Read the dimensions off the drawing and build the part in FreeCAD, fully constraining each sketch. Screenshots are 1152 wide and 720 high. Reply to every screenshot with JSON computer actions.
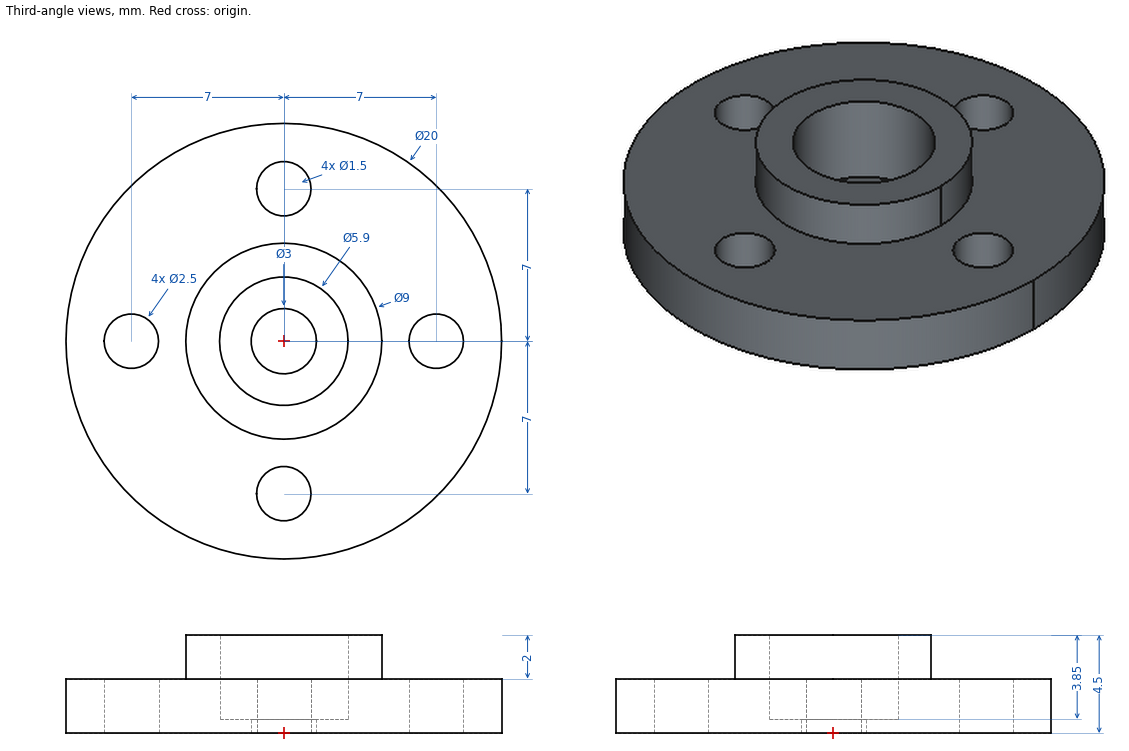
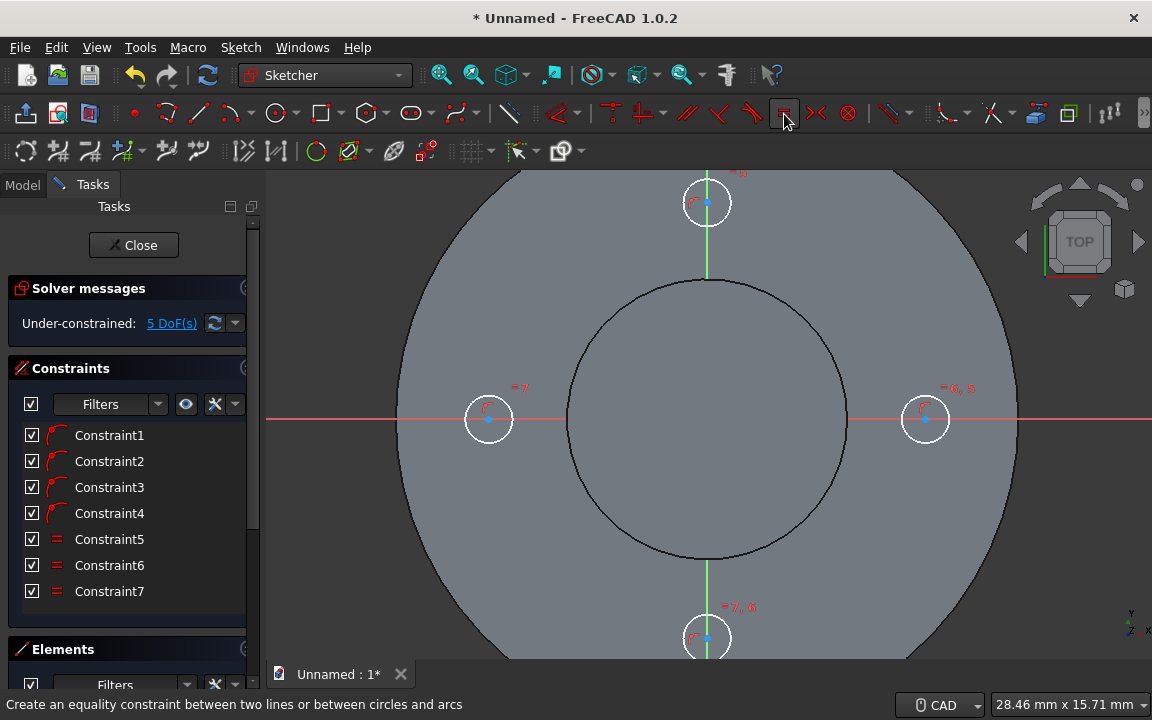
{"action": "left_click", "coordinate": [556, 114]}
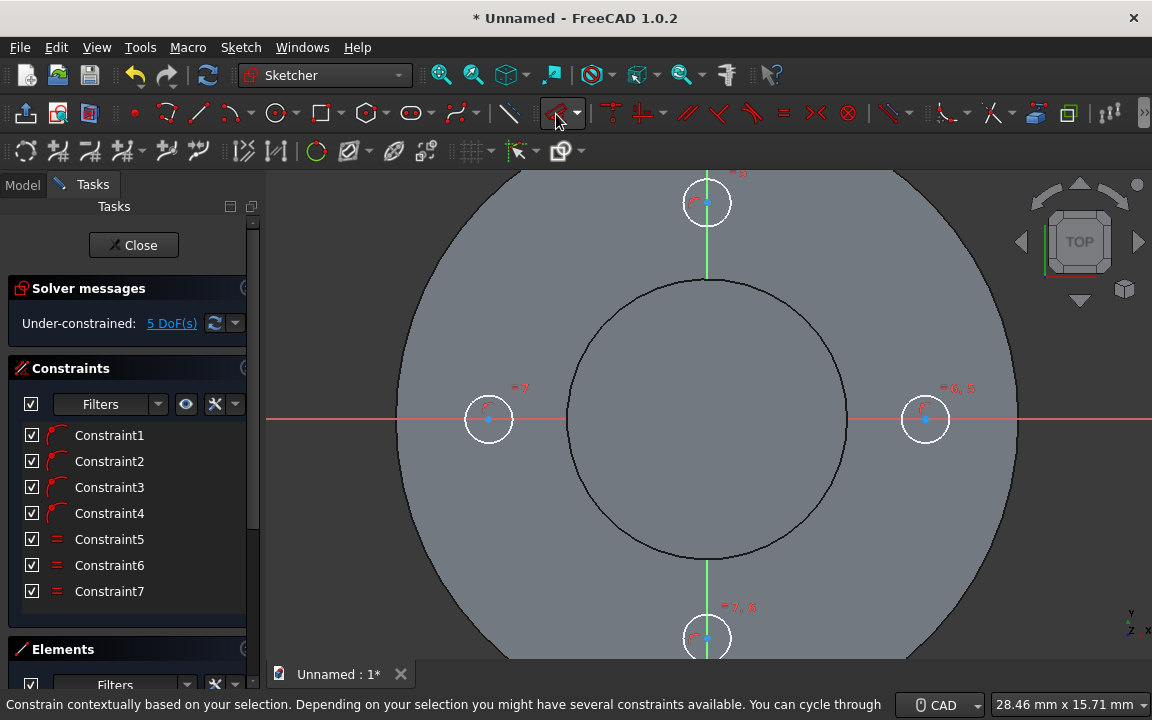
{"action": "left_click", "coordinate": [690, 220]}
{"action": "left_click", "coordinate": [667, 243]}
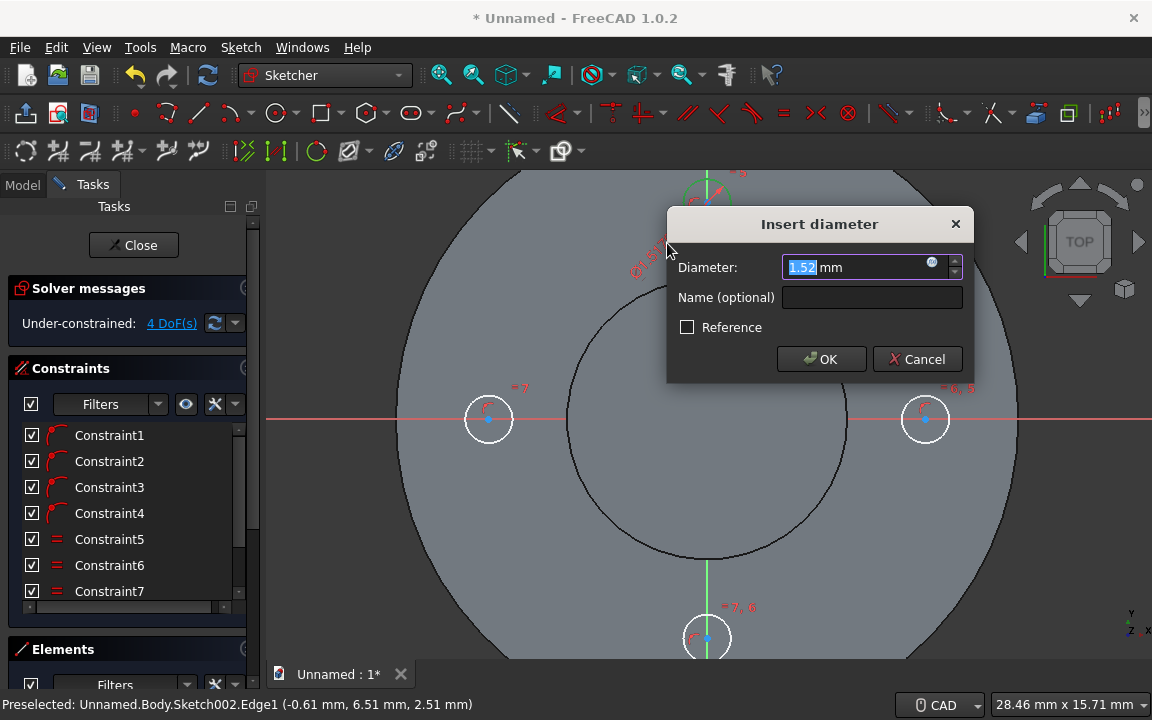
{"action": "type", "text": "1.5"}
{"action": "key", "text": "Return"}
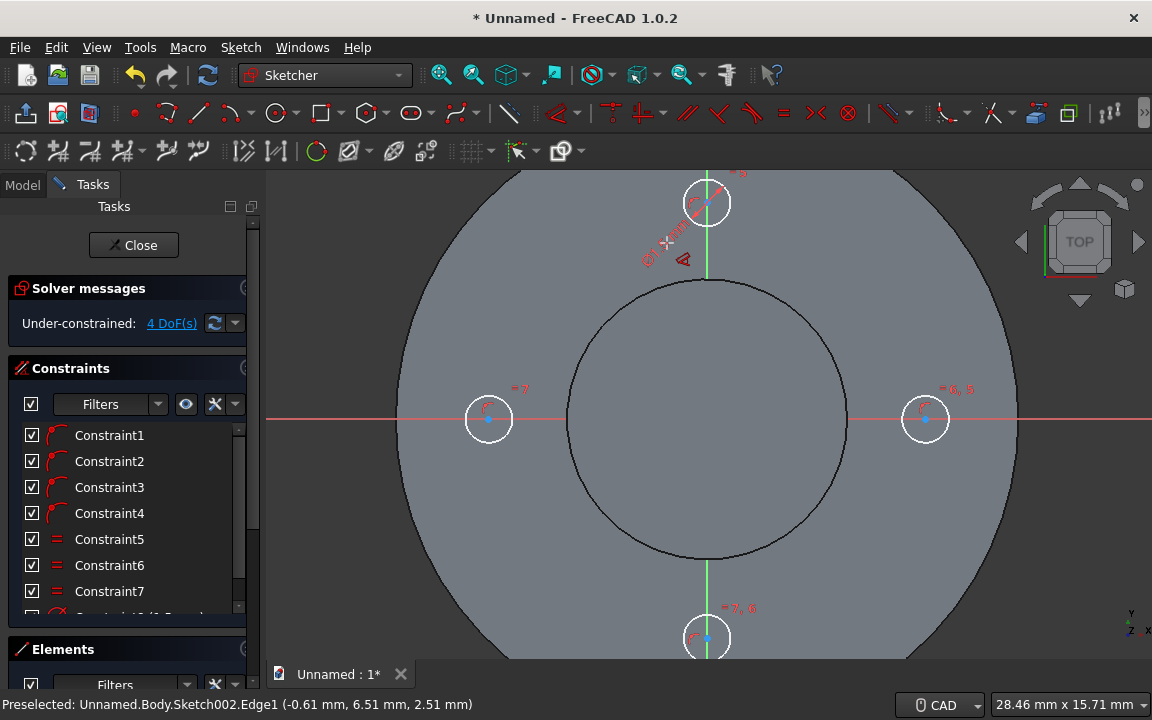
{"action": "left_click", "coordinate": [707, 203]}
{"action": "left_click", "coordinate": [741, 311]}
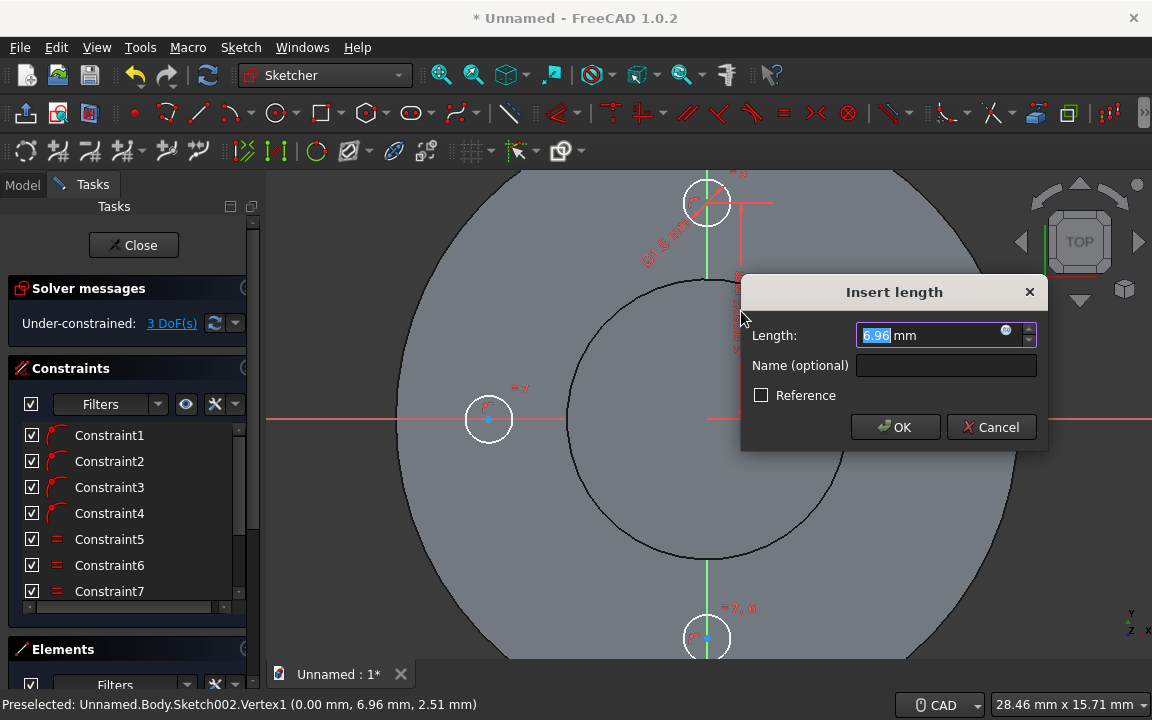
{"action": "type", "text": "7"}
{"action": "key", "text": "Return"}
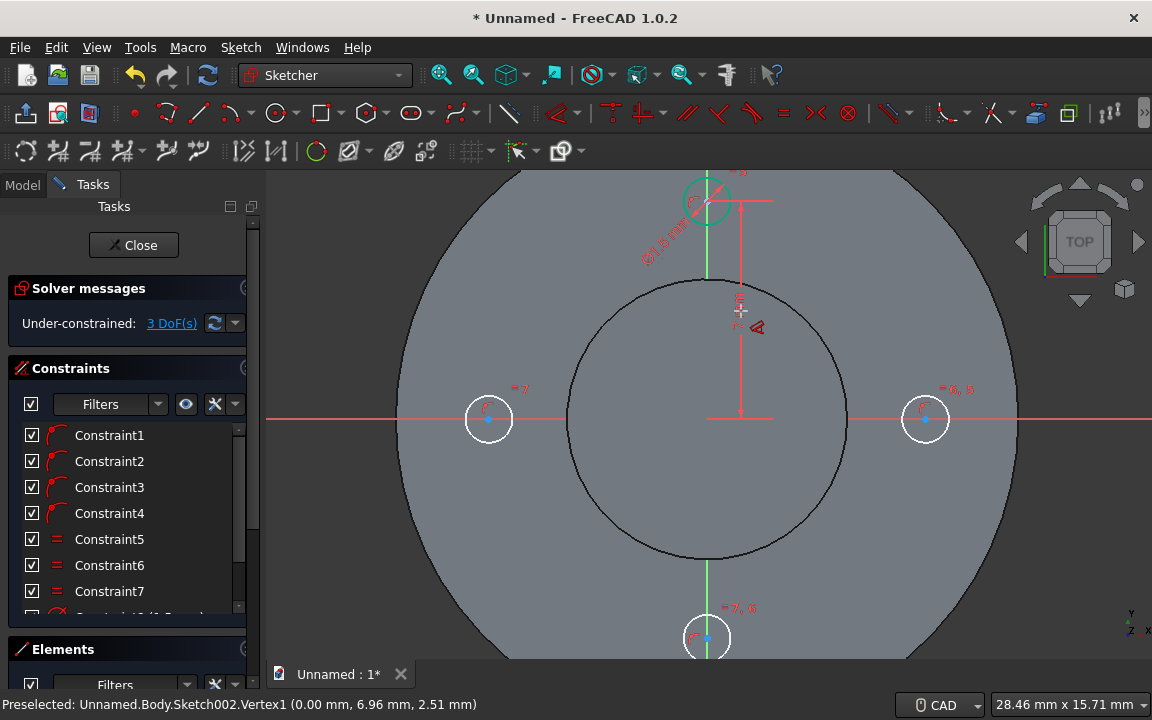
{"action": "left_click", "coordinate": [926, 419]}
{"action": "left_click", "coordinate": [816, 453]}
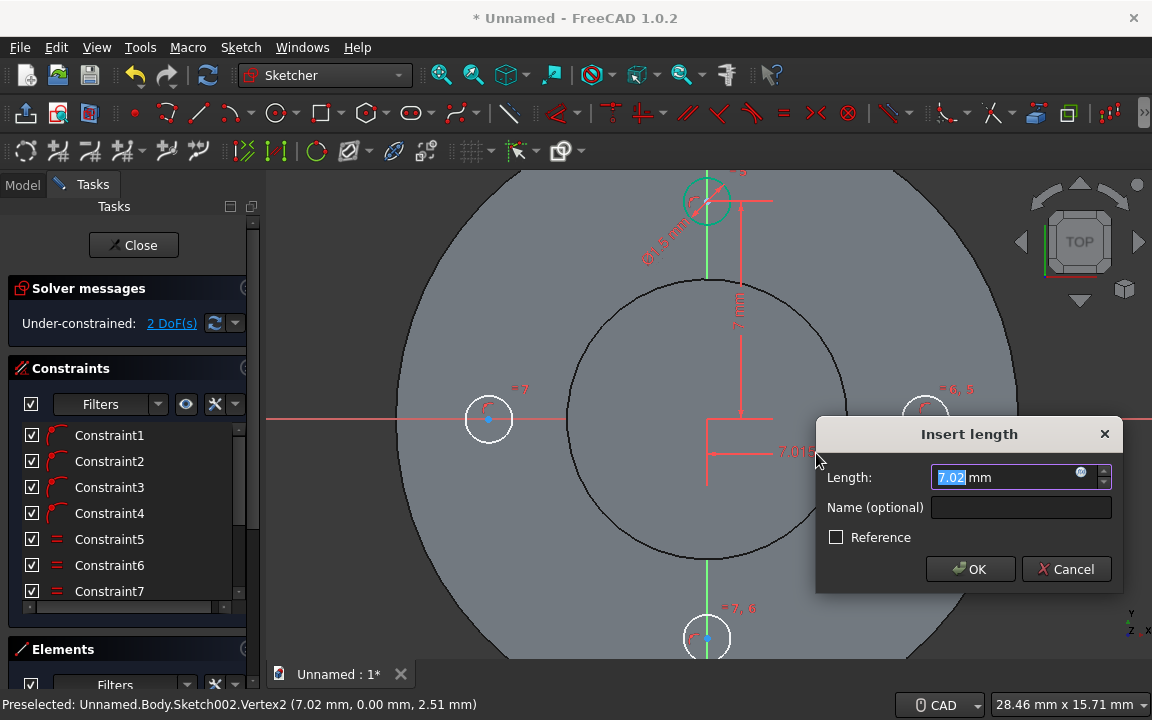
{"action": "type", "text": "7"}
{"action": "key", "text": "Return"}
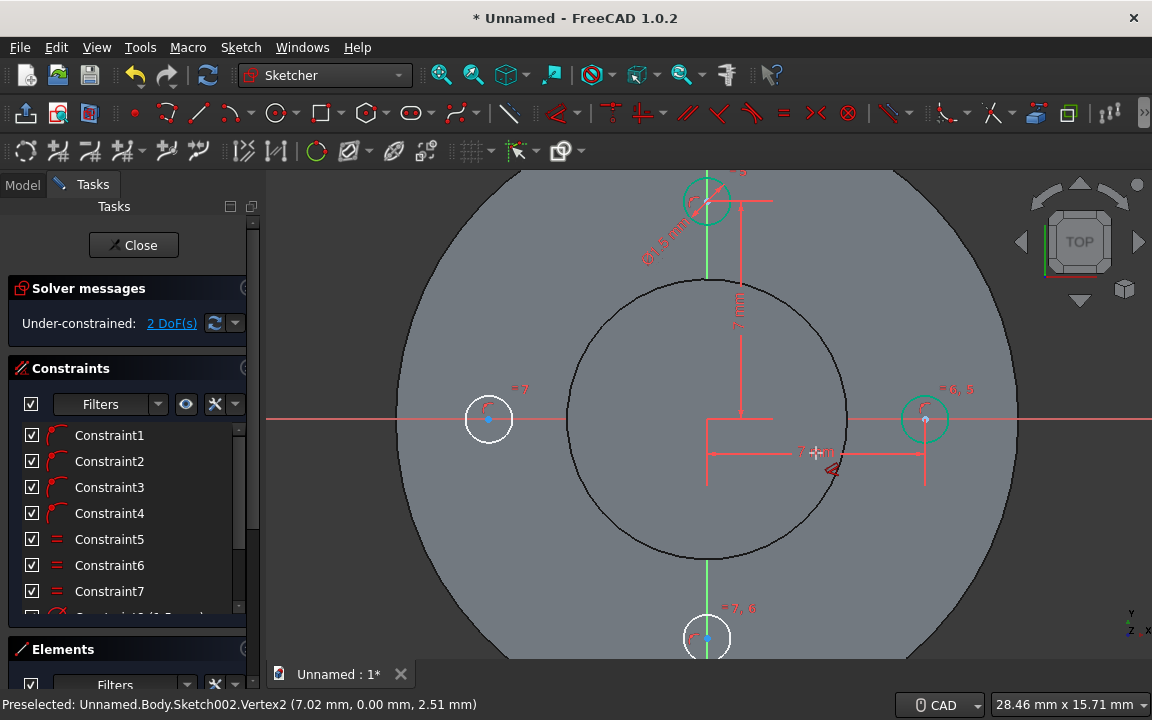
{"action": "scroll", "coordinate": [505, 405], "scroll_direction": "down", "scroll_amount": 2}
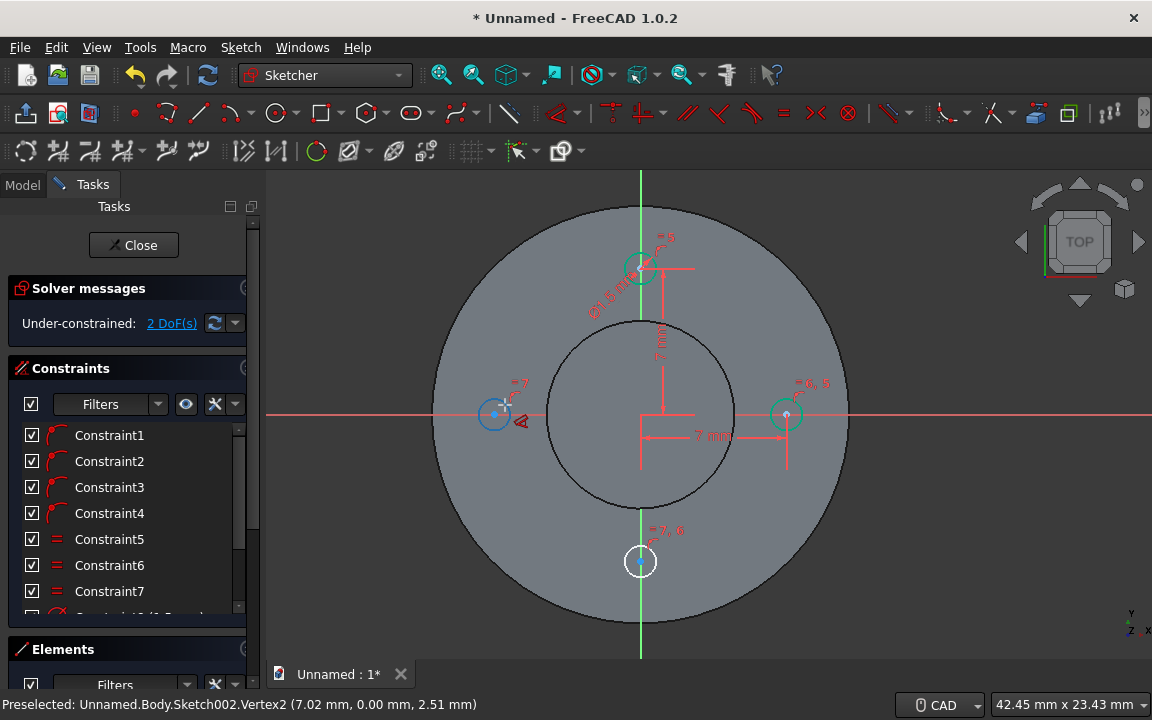
{"action": "left_click", "coordinate": [641, 562]}
{"action": "left_click", "coordinate": [675, 488]}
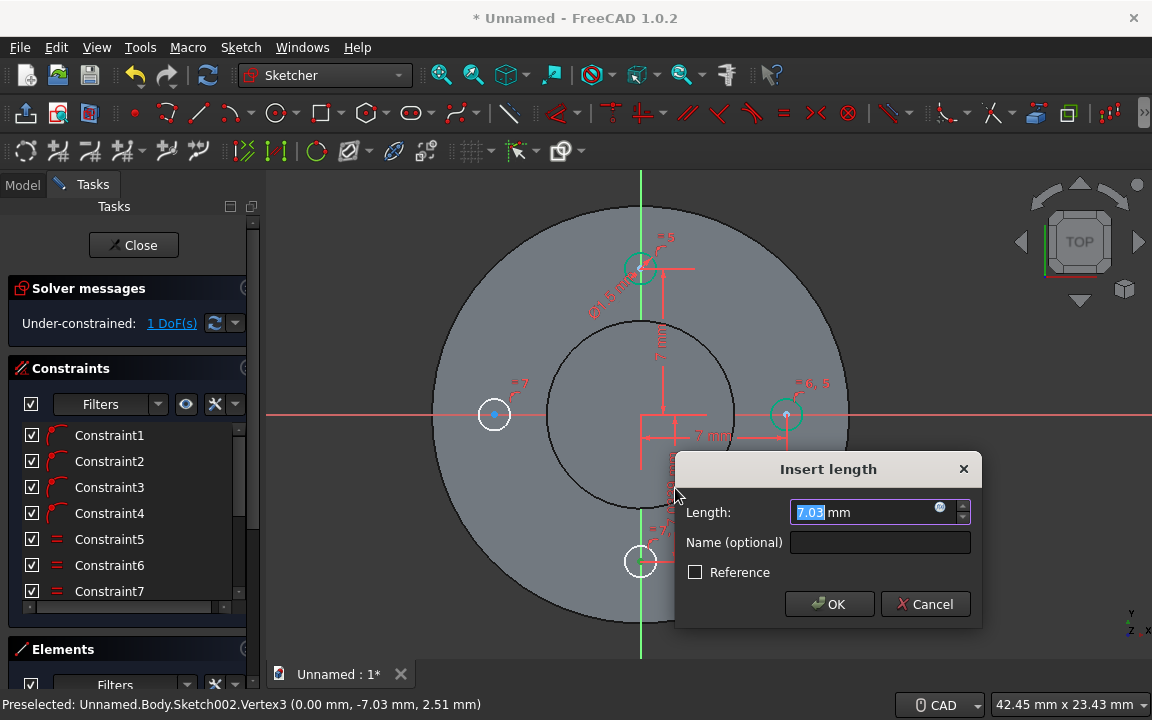
{"action": "type", "text": "7"}
{"action": "key", "text": "Return"}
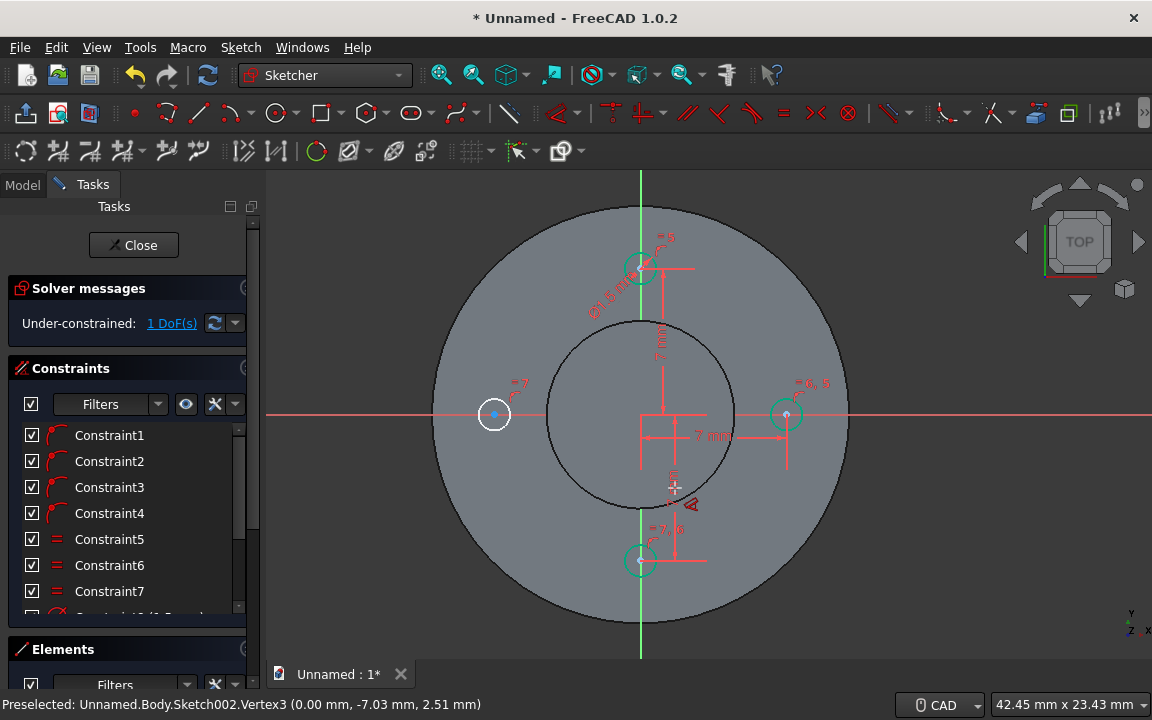
{"action": "left_click", "coordinate": [494, 415]}
{"action": "left_click", "coordinate": [567, 449]}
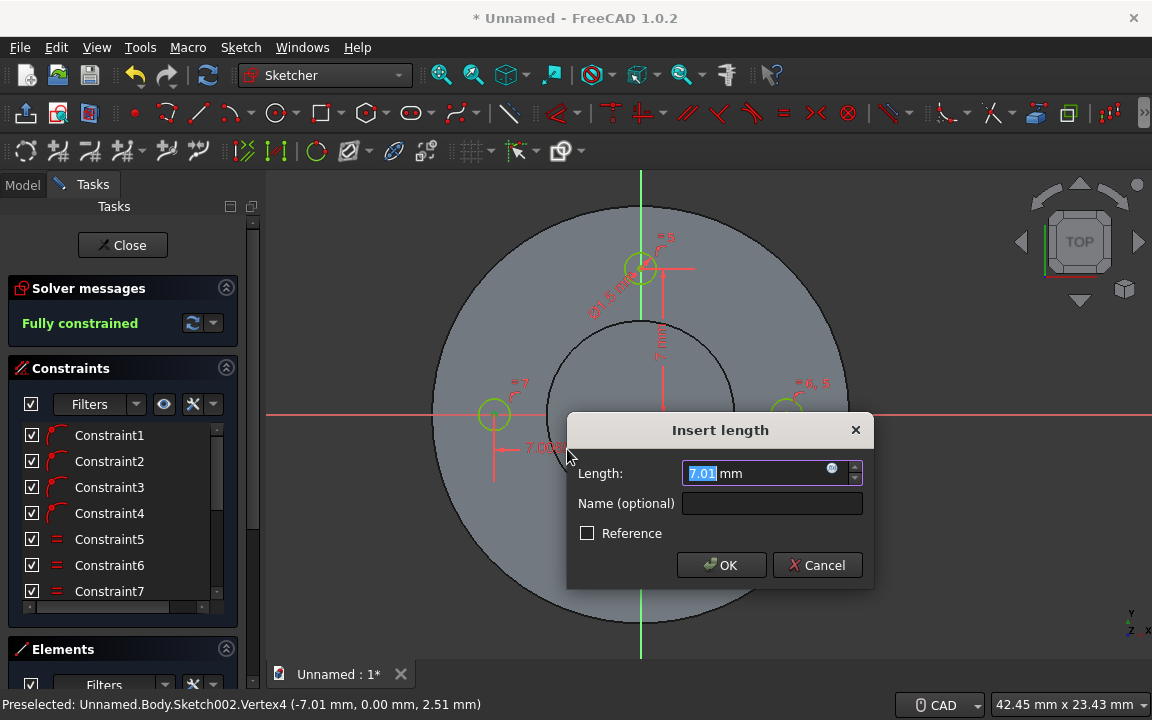
{"action": "type", "text": "7"}
{"action": "key", "text": "Return"}
{"action": "key", "text": "Escape"}